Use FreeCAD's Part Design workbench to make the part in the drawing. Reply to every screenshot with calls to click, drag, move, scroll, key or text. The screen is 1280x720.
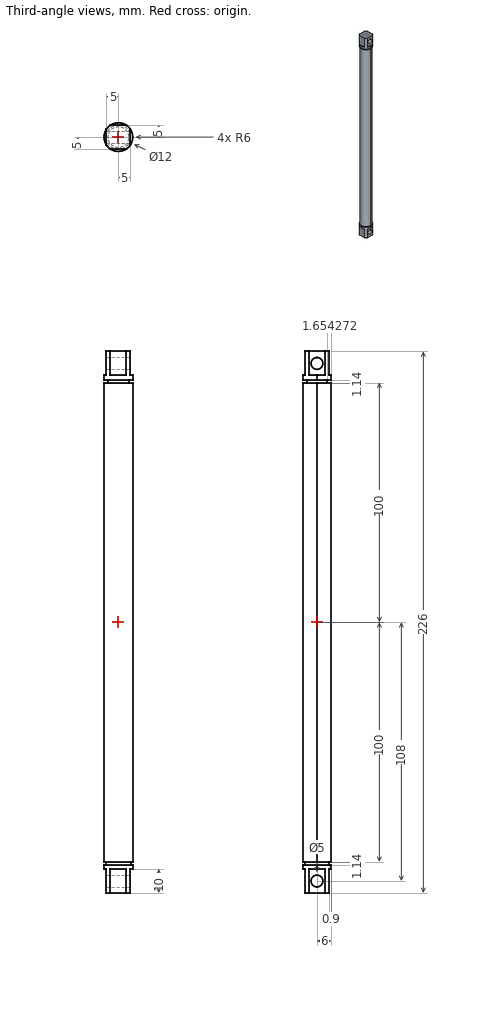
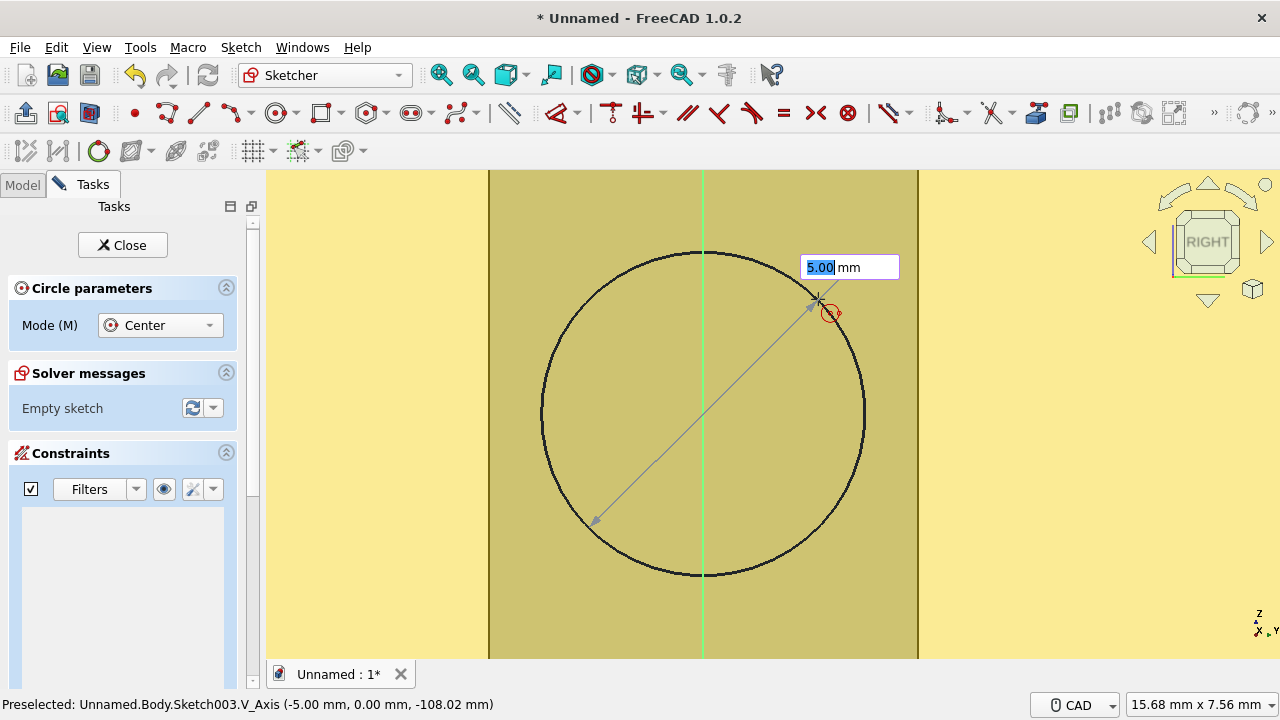
text(5)
key(Return)
key(Escape)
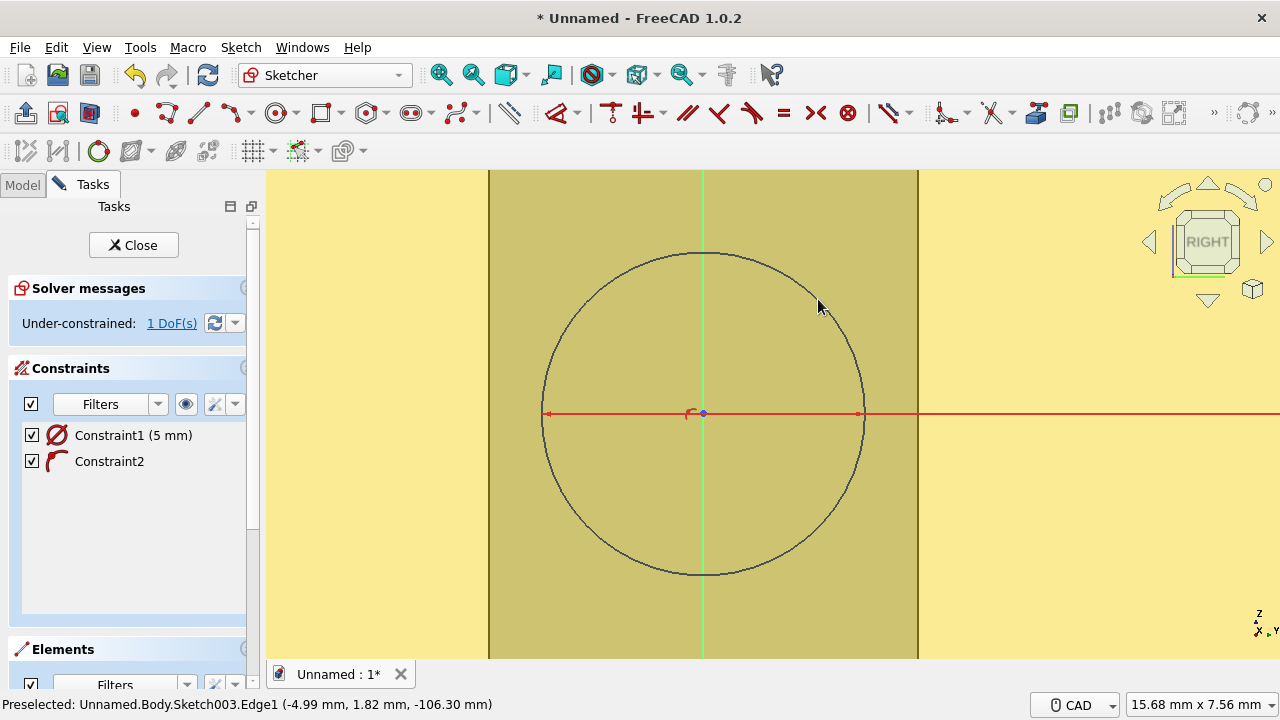
key(d)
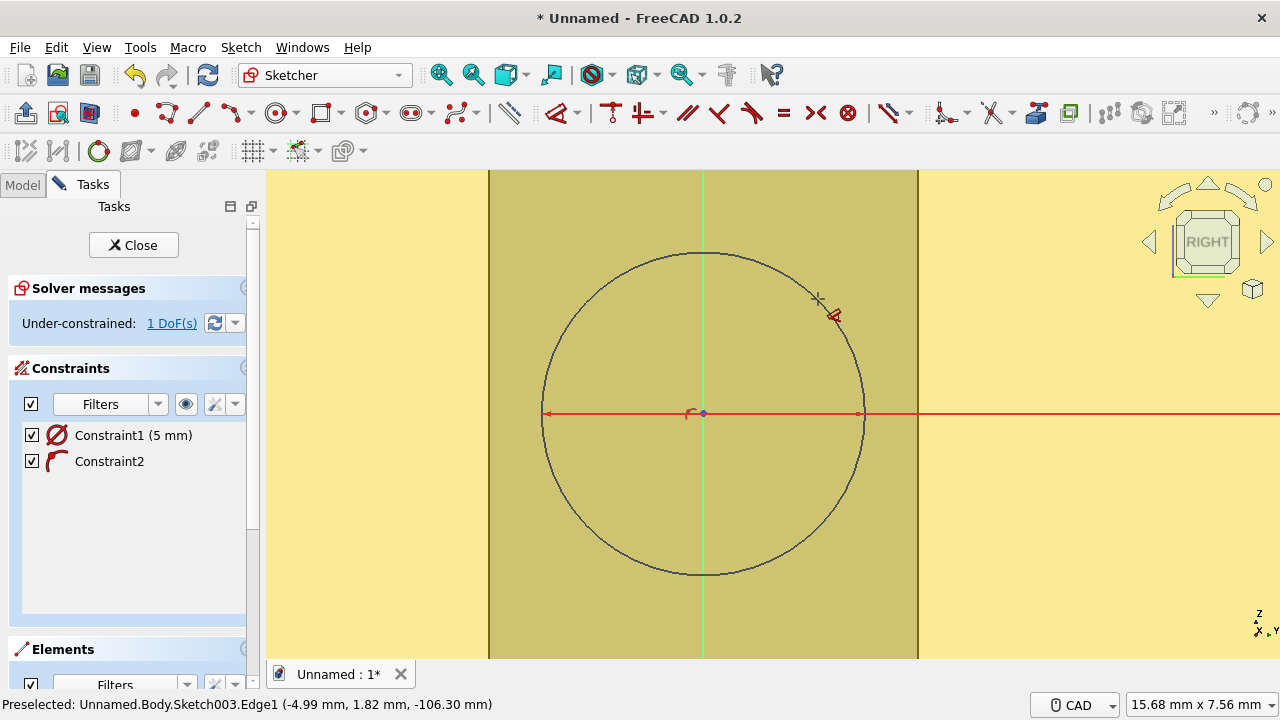
click(703, 414)
click(737, 306)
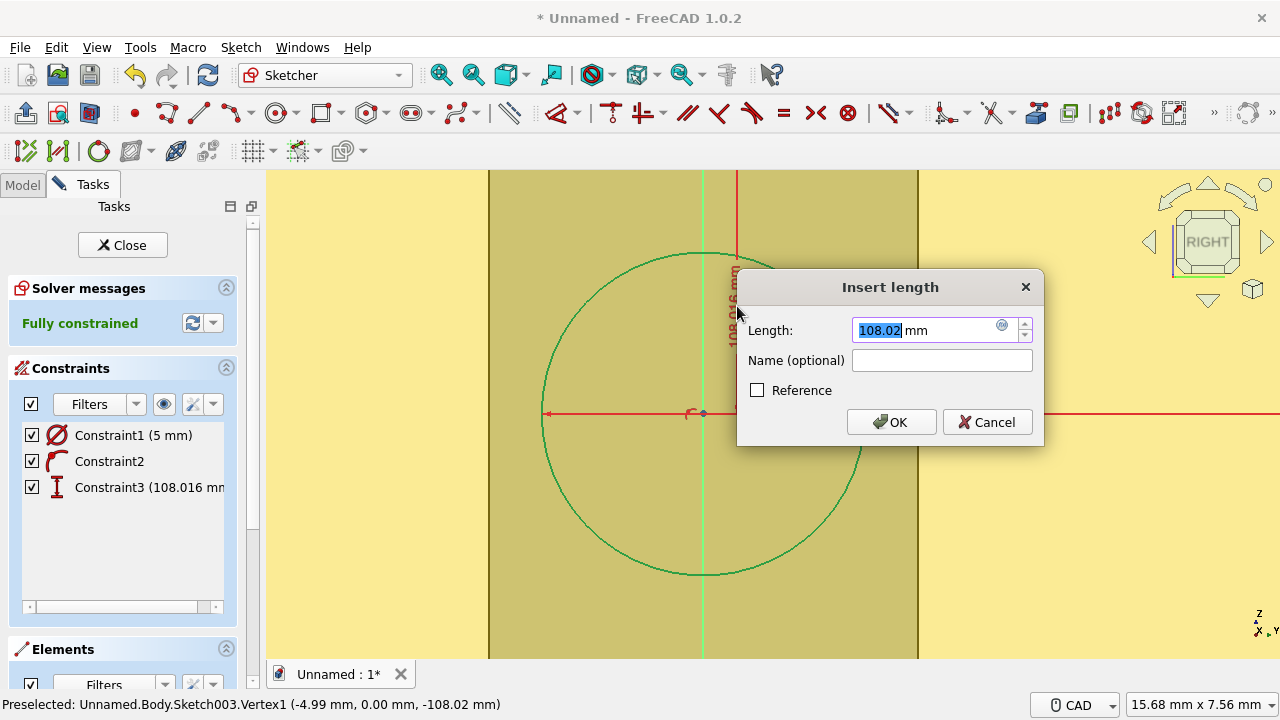
text(108)
key(Return)
key(Escape)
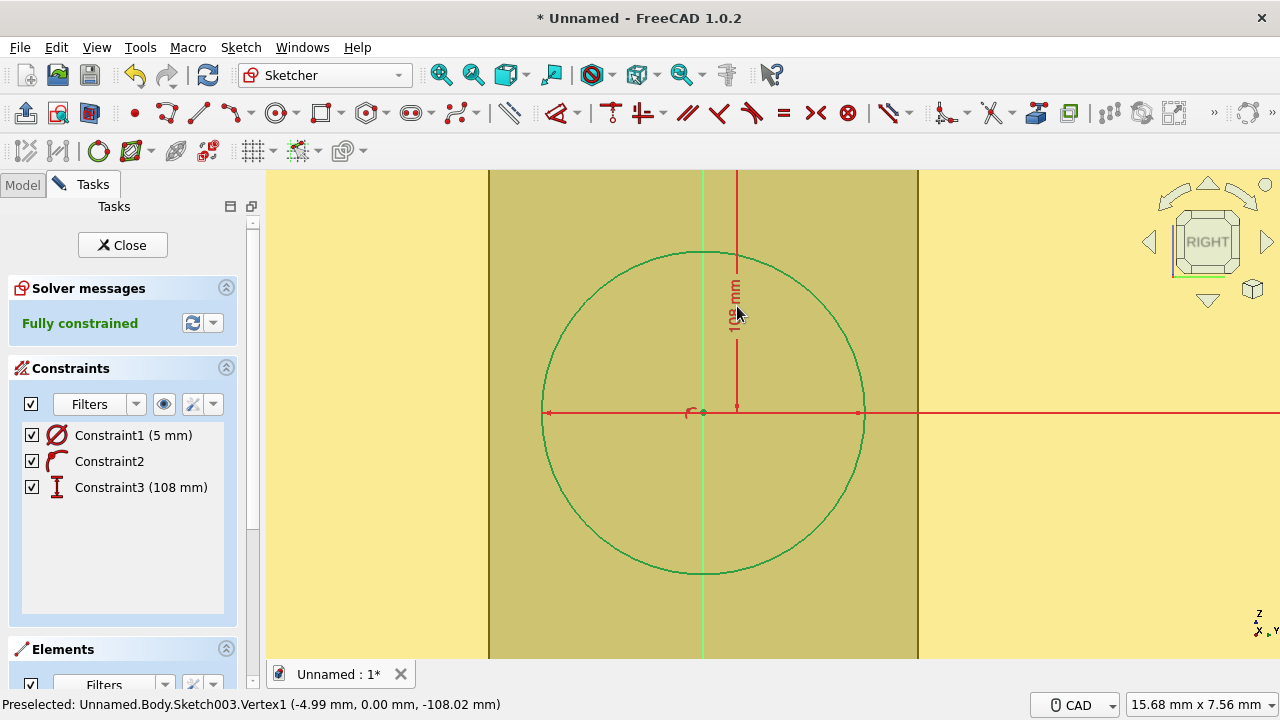
click(123, 245)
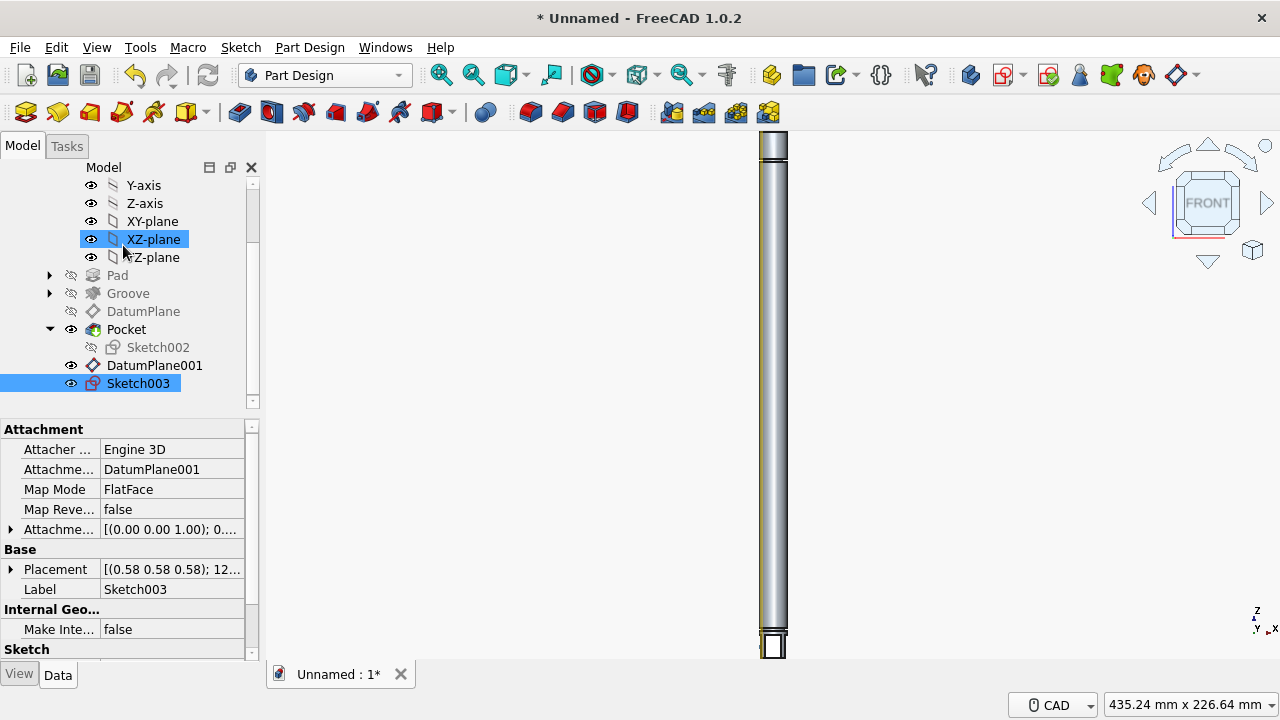
click(240, 112)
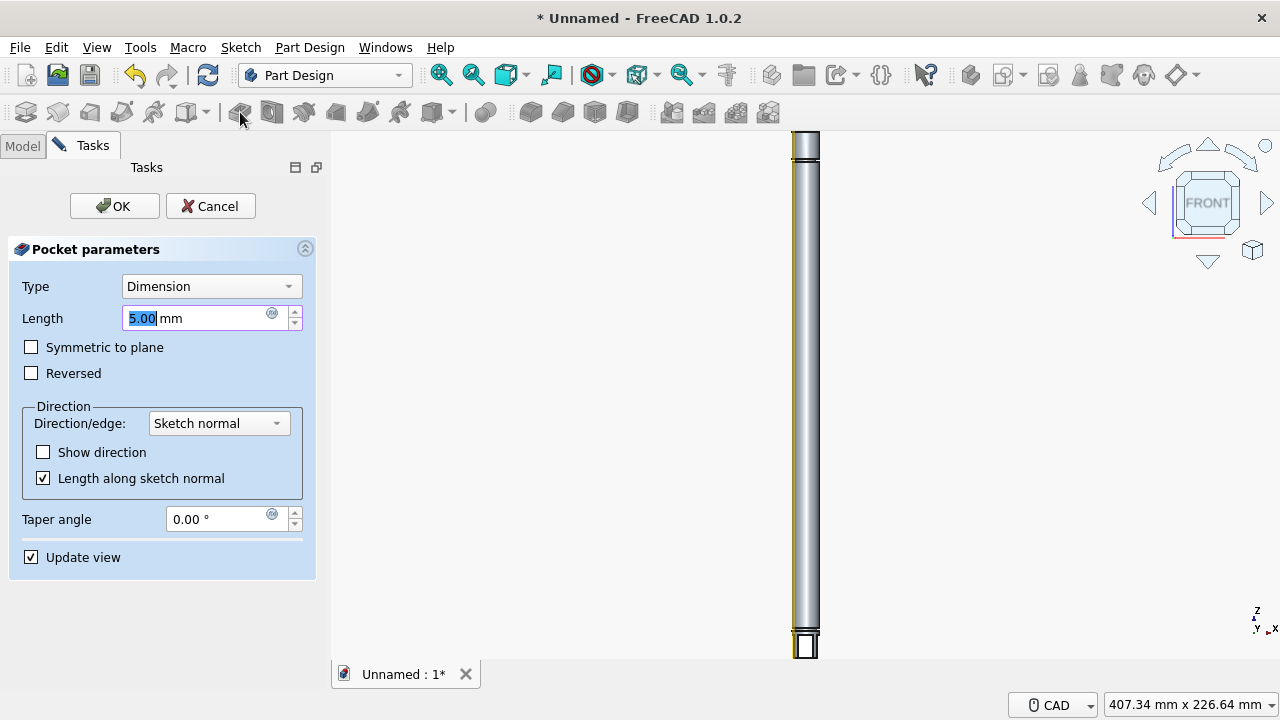
click(212, 286)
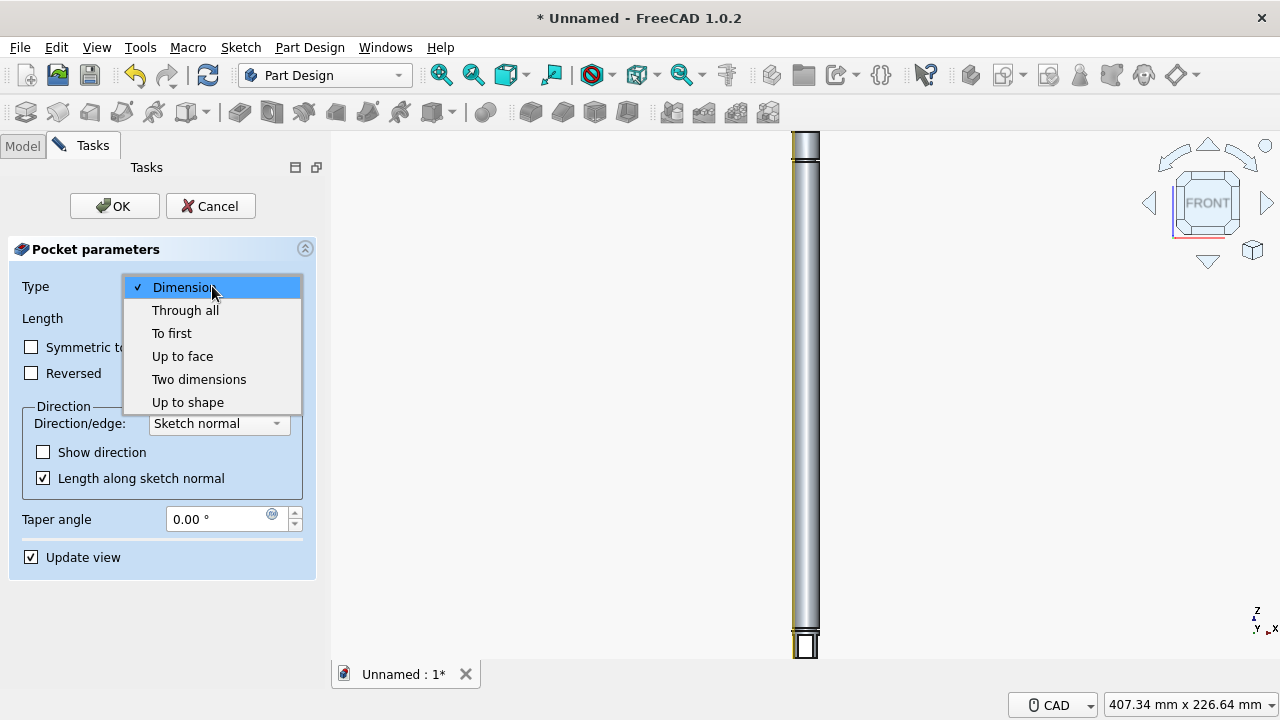
click(212, 310)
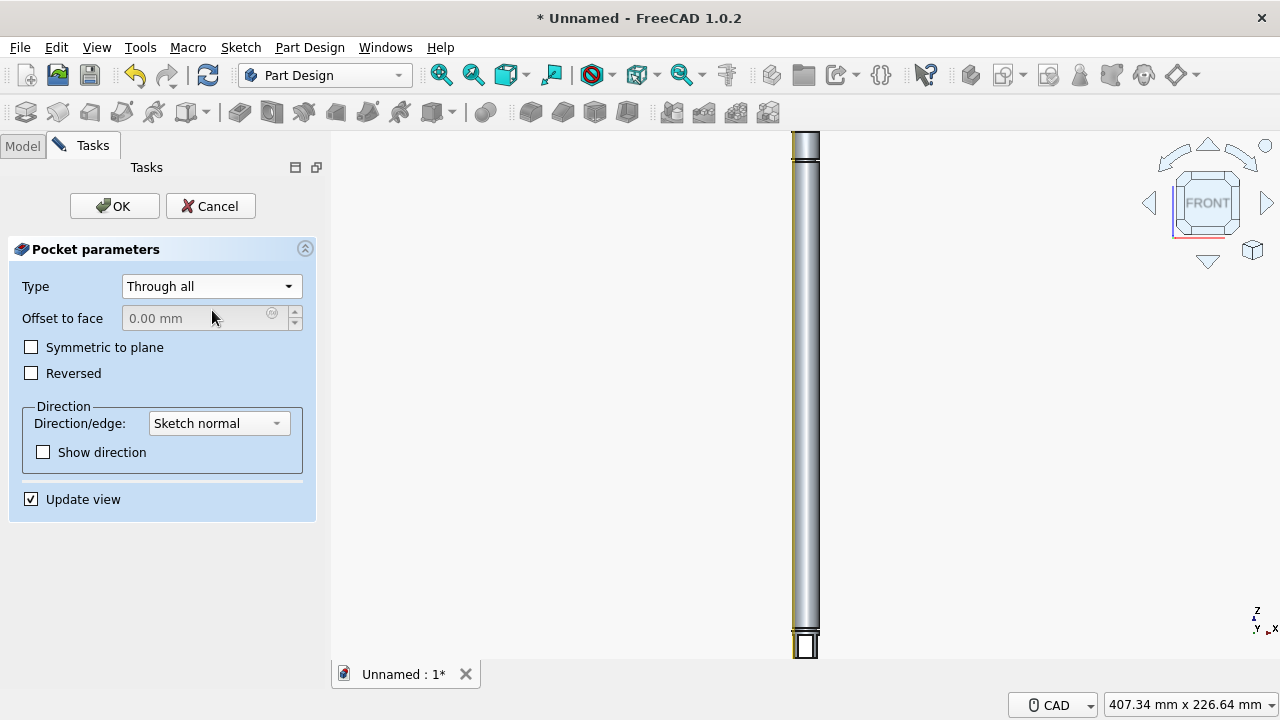
click(30, 373)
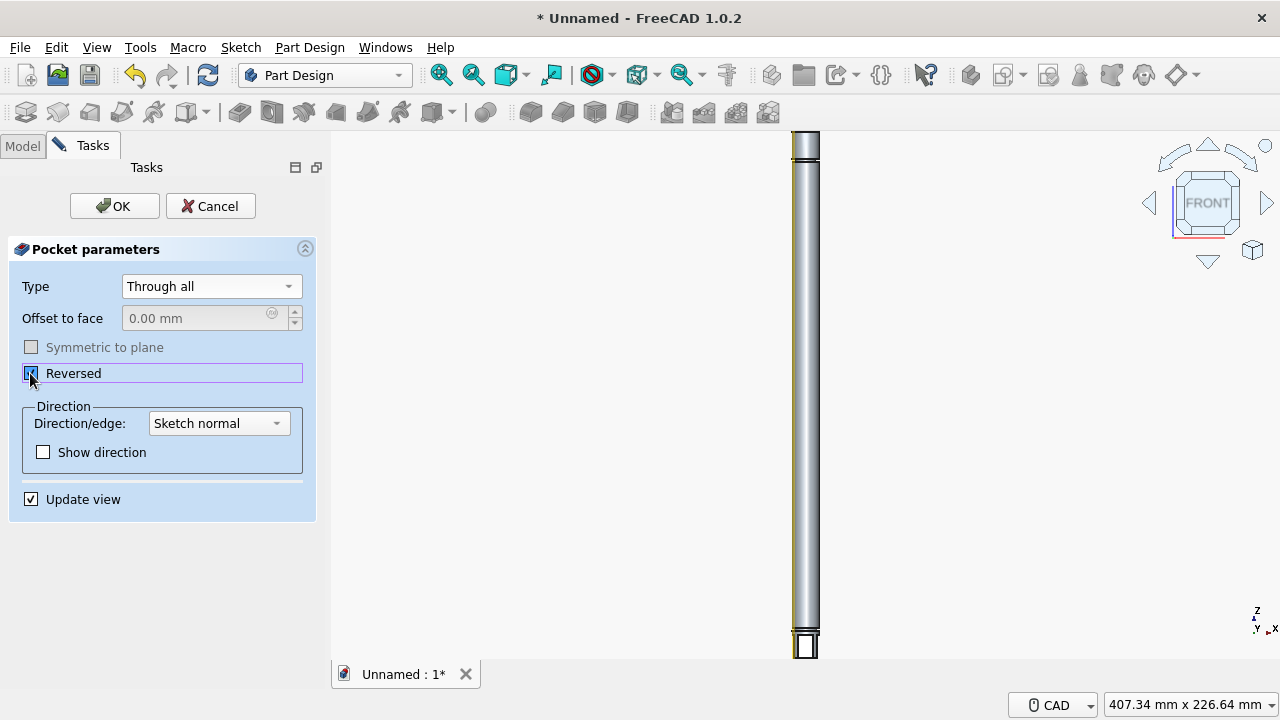
click(115, 206)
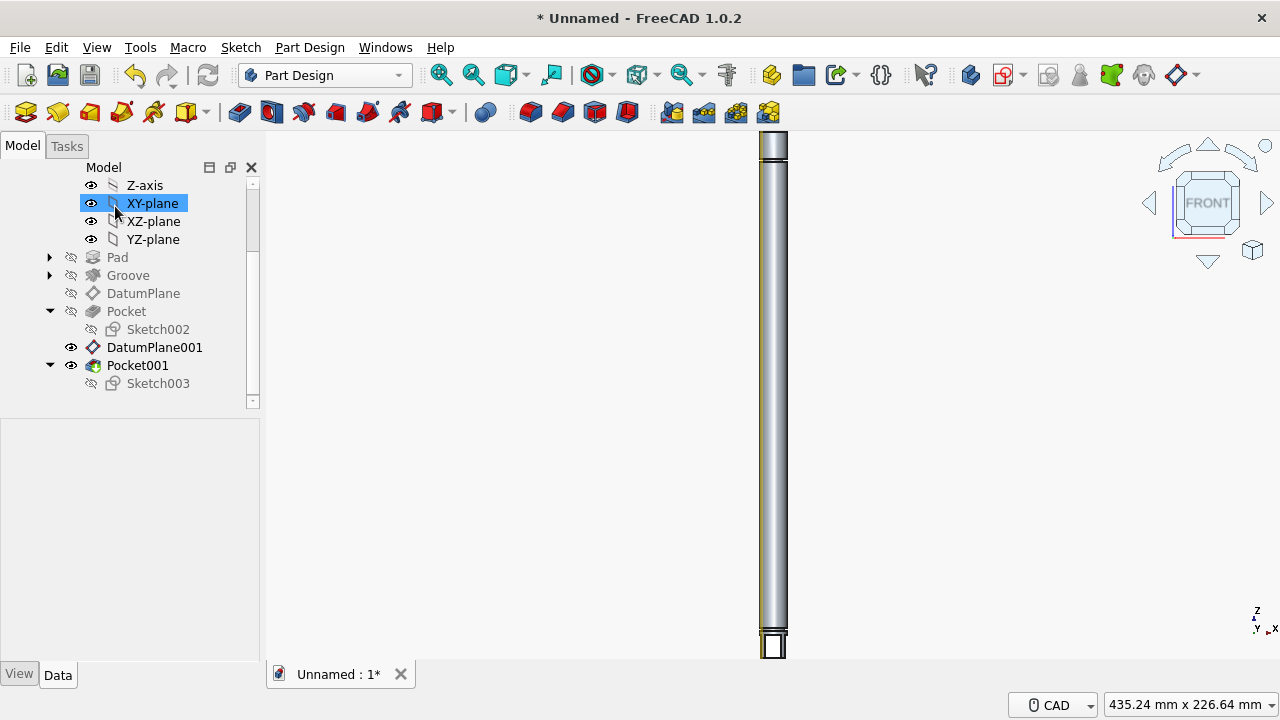
click(116, 347)
key(space)